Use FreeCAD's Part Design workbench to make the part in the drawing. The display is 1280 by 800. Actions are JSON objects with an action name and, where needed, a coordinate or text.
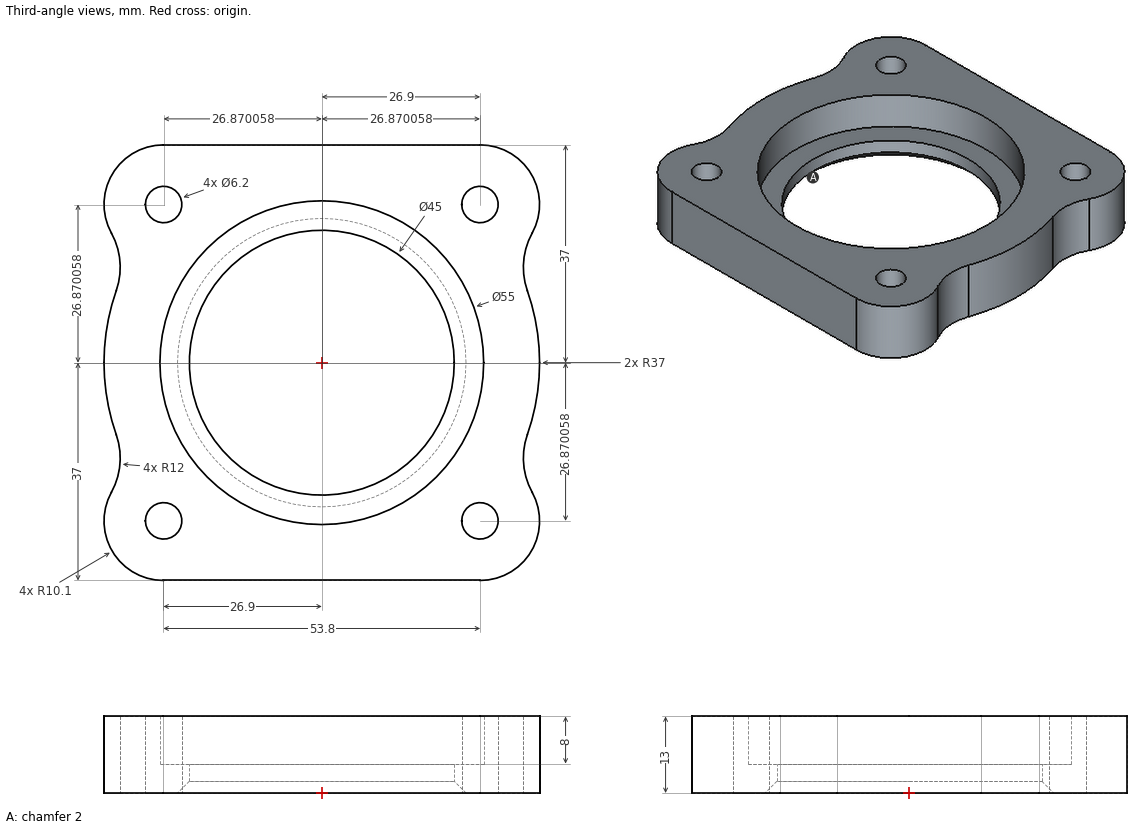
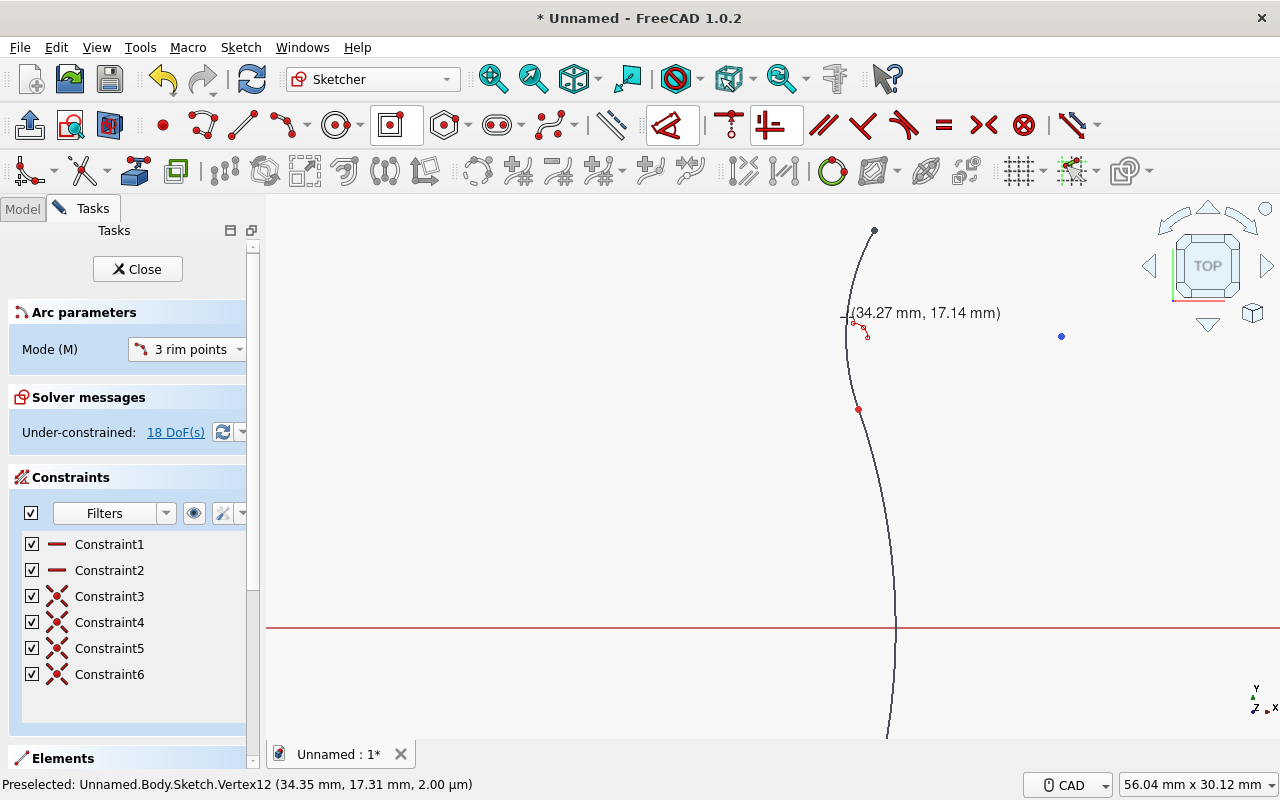
{"action": "left_click", "coordinate": [874, 231]}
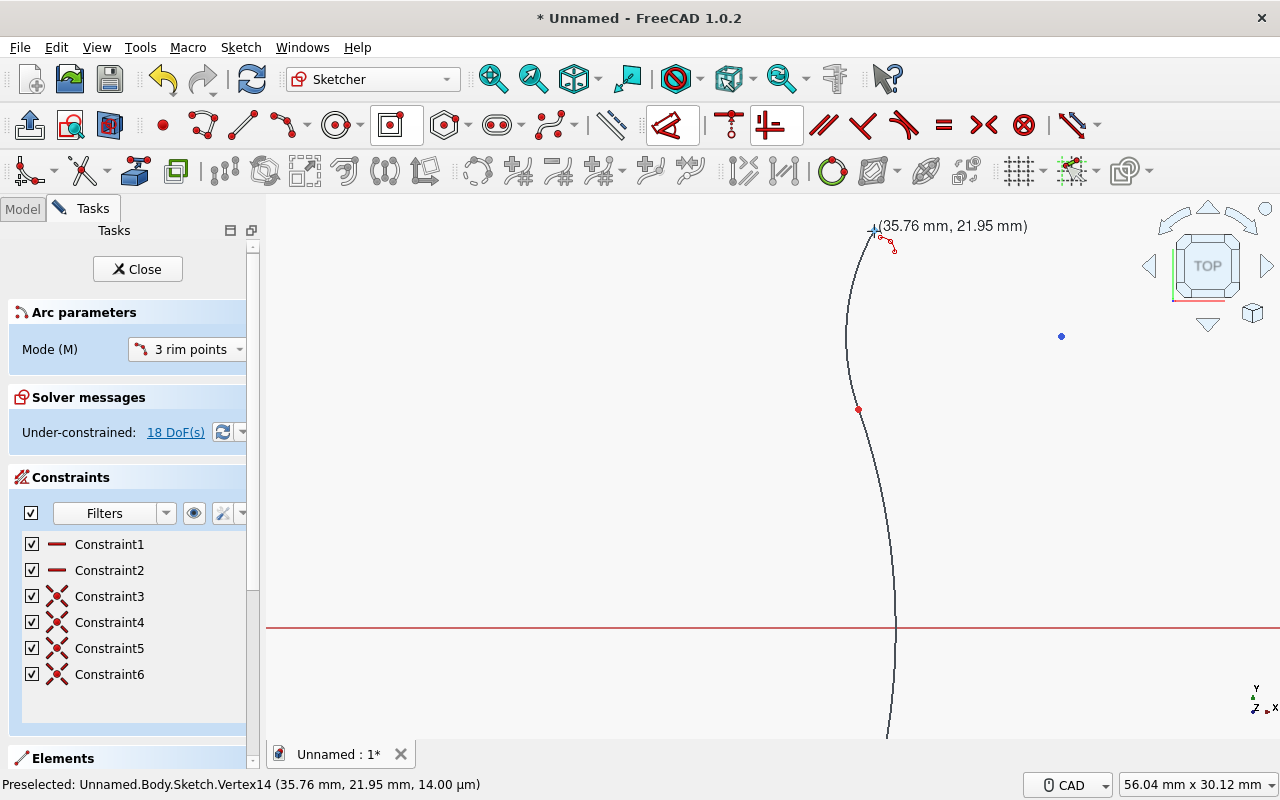
{"action": "scroll", "coordinate": [861, 414], "scroll_direction": "down", "scroll_amount": 7}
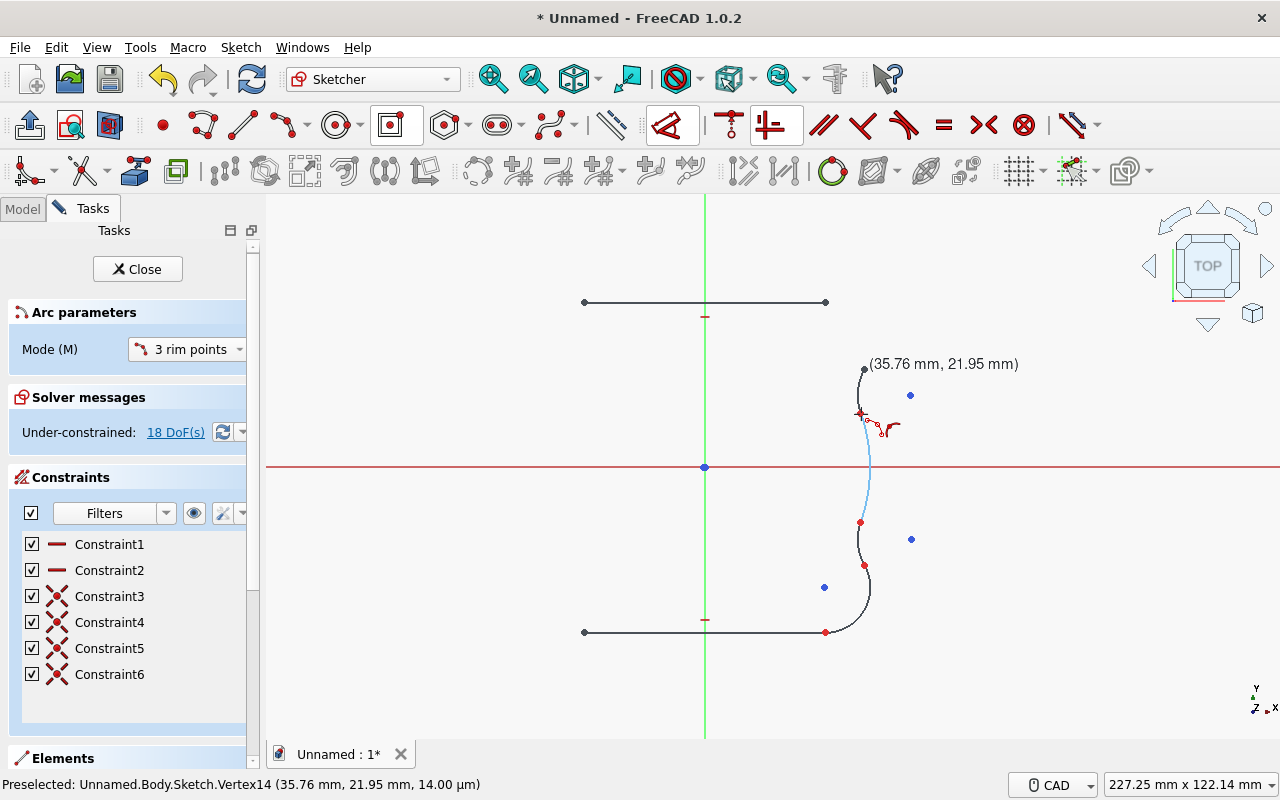
{"action": "left_click", "coordinate": [825, 303]}
{"action": "left_click", "coordinate": [864, 324]}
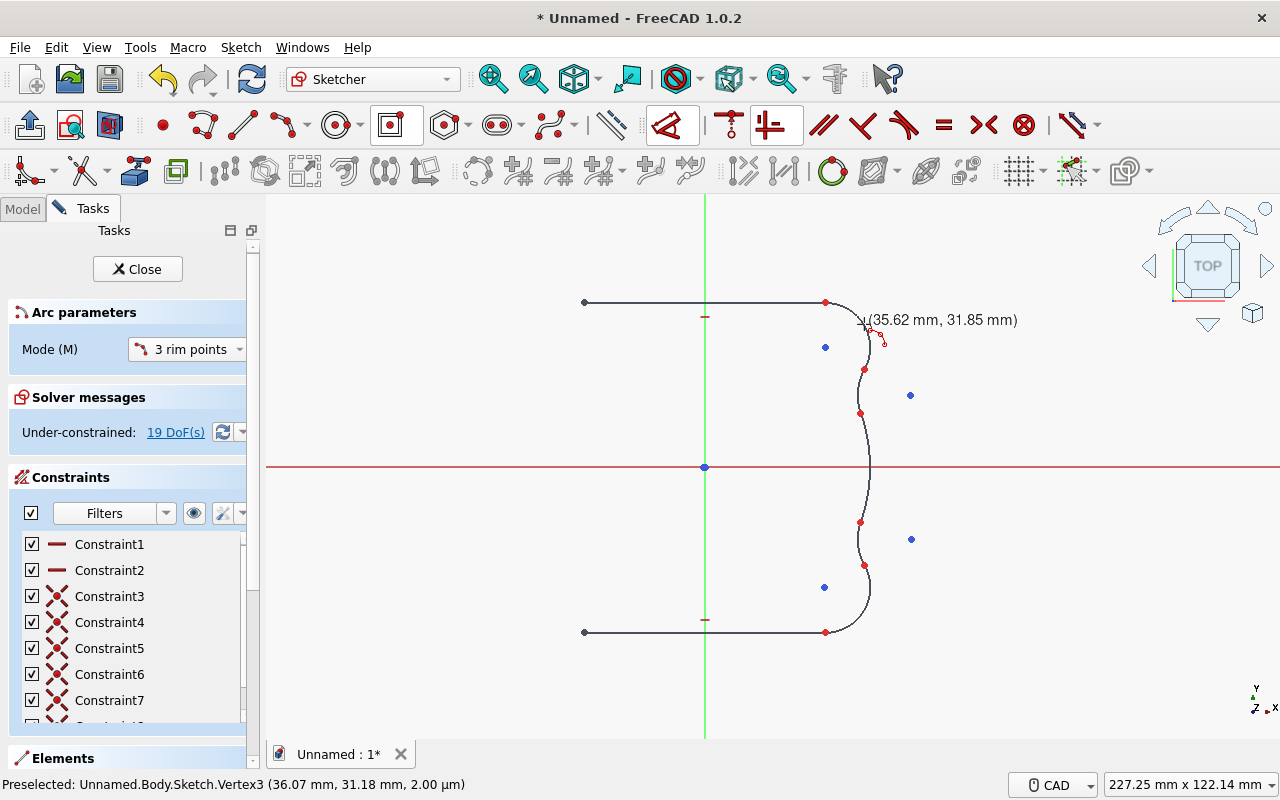
{"action": "left_click", "coordinate": [585, 303]}
{"action": "left_click", "coordinate": [546, 369]}
{"action": "left_click", "coordinate": [546, 324]}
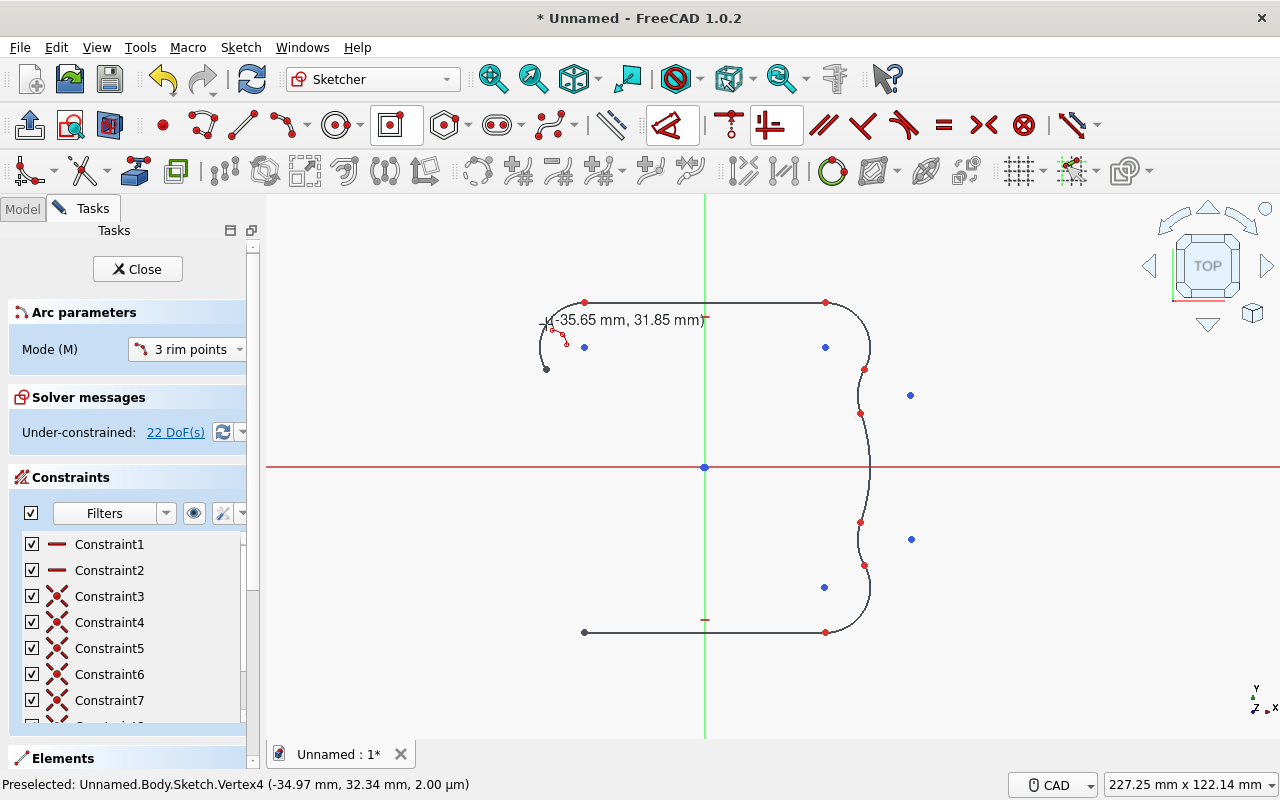
{"action": "left_click", "coordinate": [546, 370]}
{"action": "left_click", "coordinate": [549, 412]}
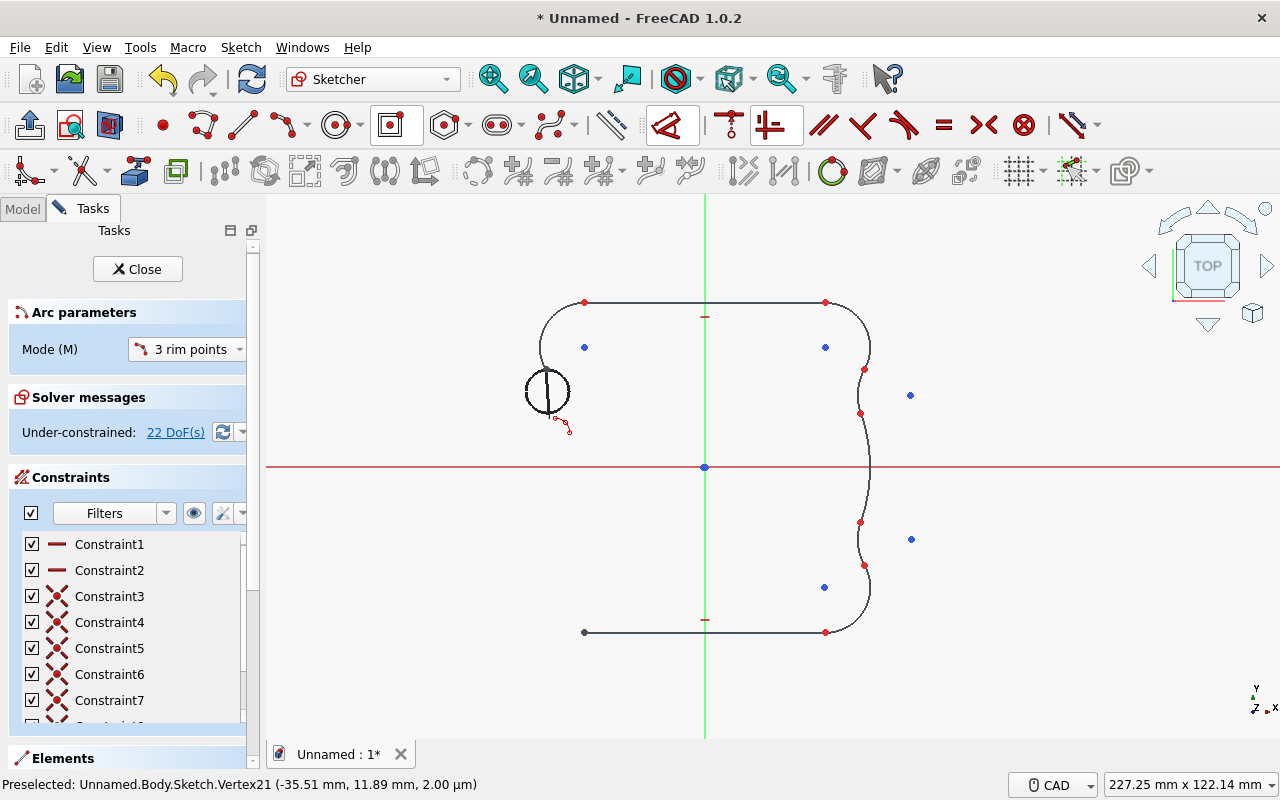
{"action": "scroll", "coordinate": [552, 390], "scroll_direction": "up", "scroll_amount": 7}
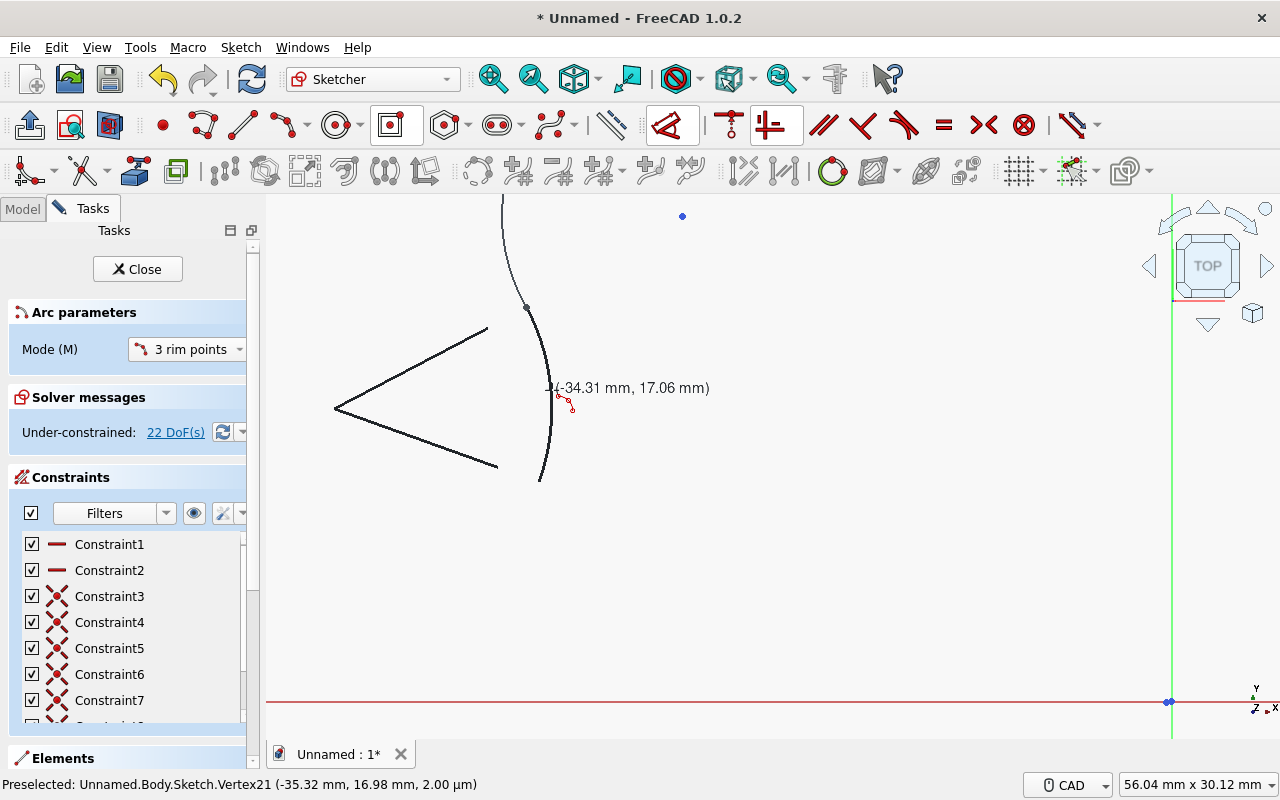
{"action": "left_click", "coordinate": [552, 390]}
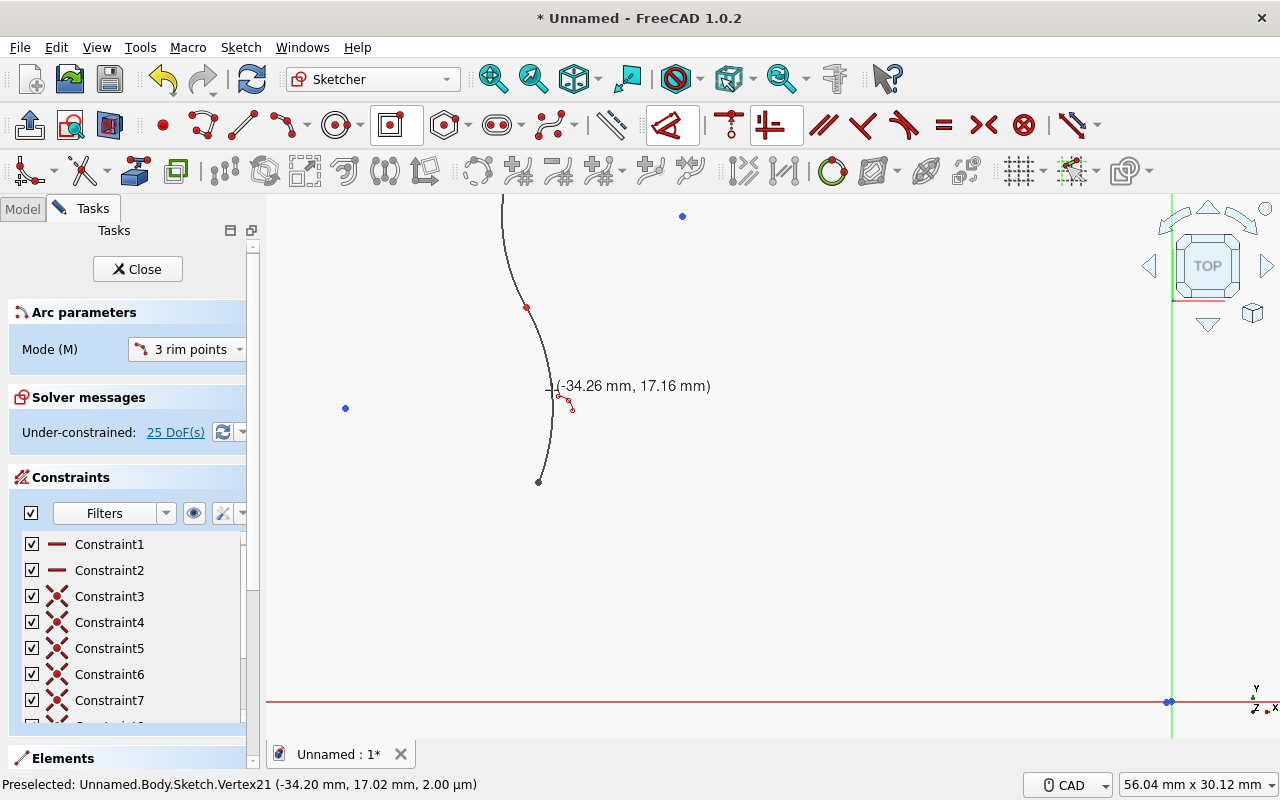
{"action": "left_click", "coordinate": [539, 482]}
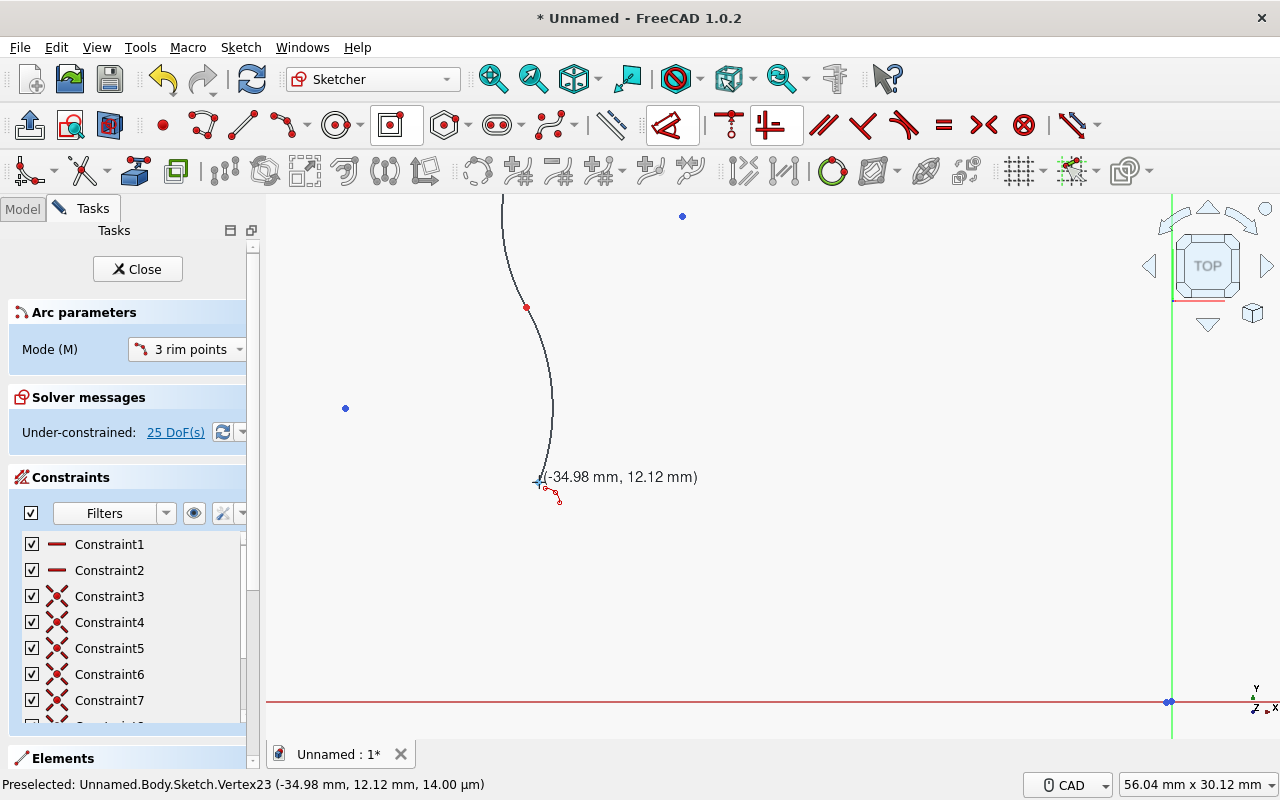
{"action": "scroll", "coordinate": [552, 390], "scroll_direction": "down", "scroll_amount": 7}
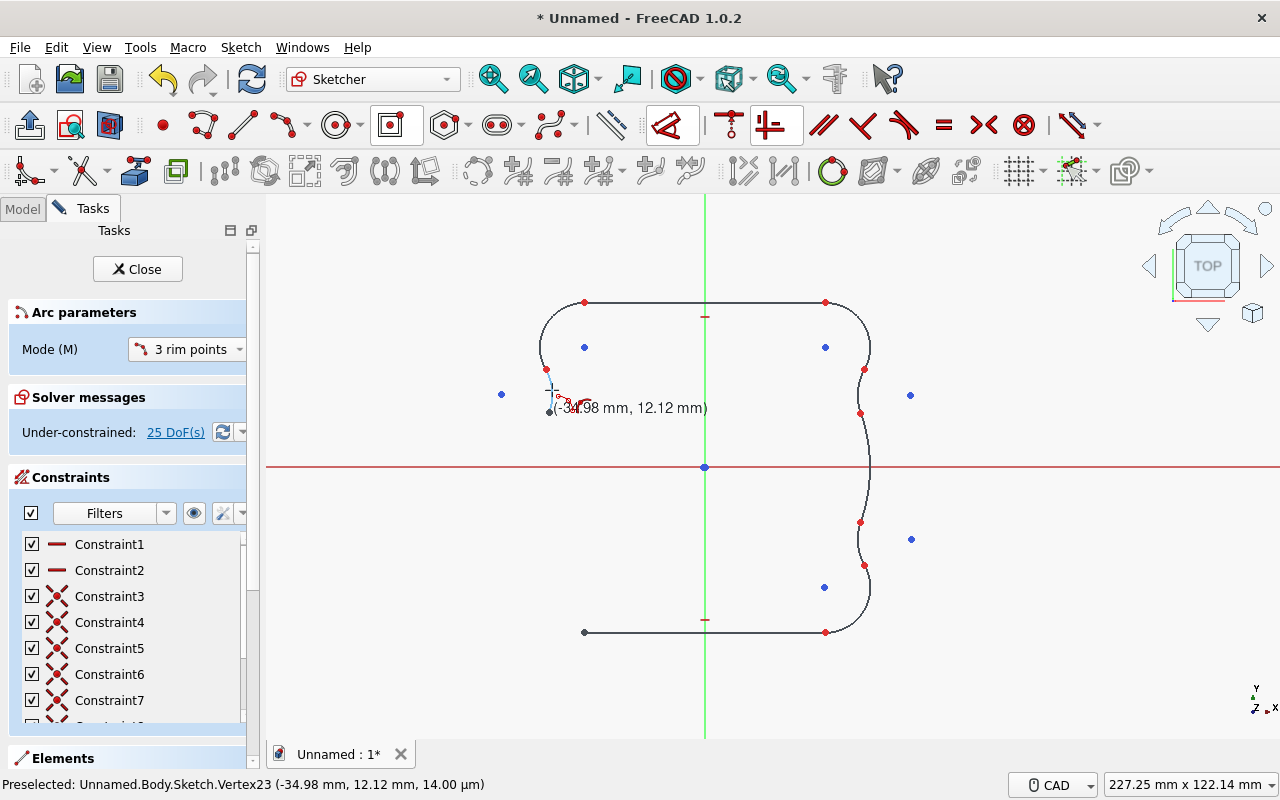
{"action": "left_click", "coordinate": [549, 522]}